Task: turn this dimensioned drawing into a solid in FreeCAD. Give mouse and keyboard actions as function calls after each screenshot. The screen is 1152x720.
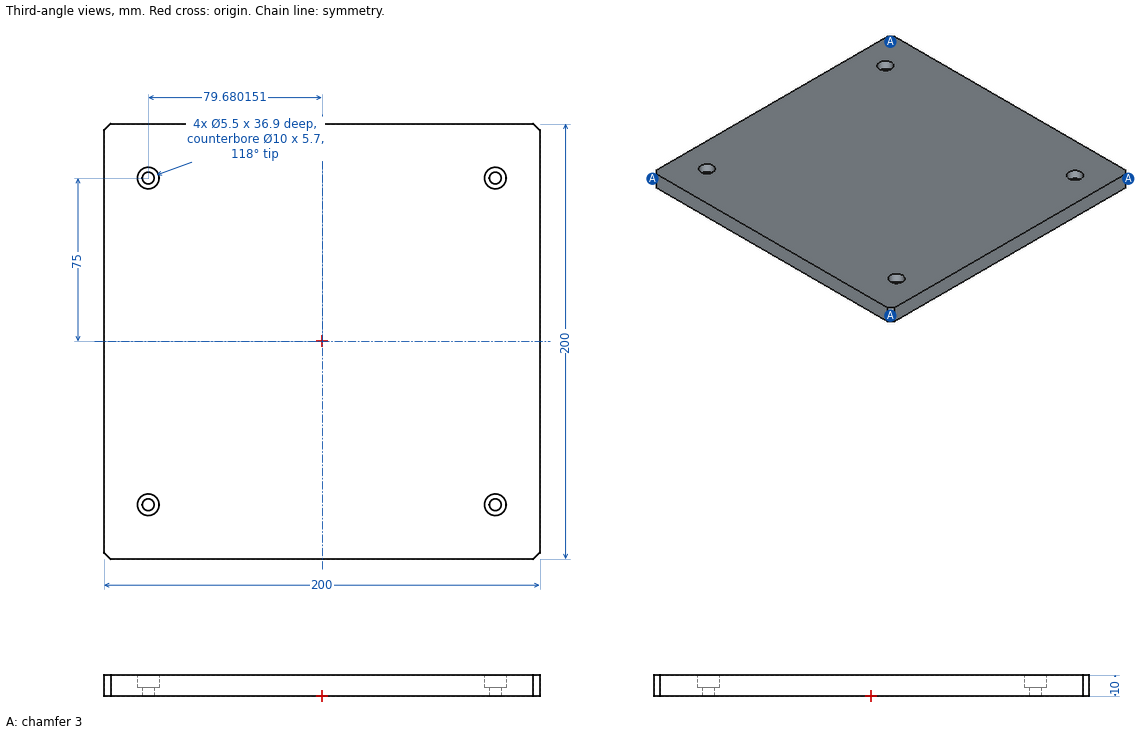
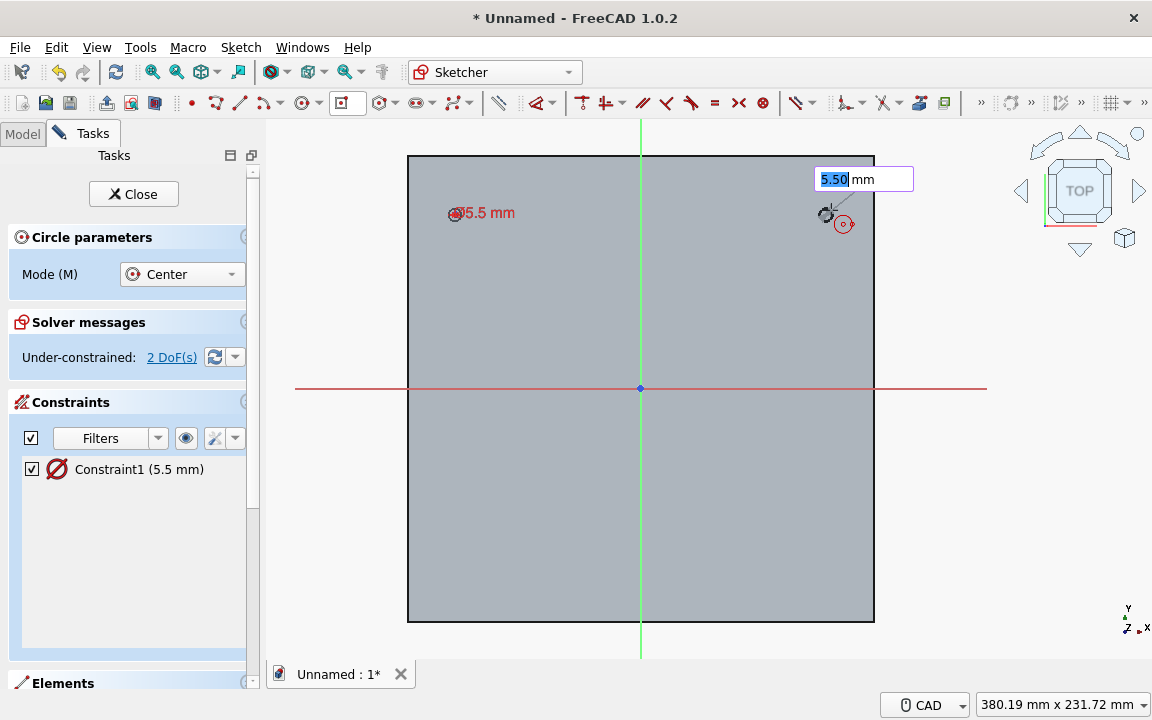
text(5.5)
key(Return)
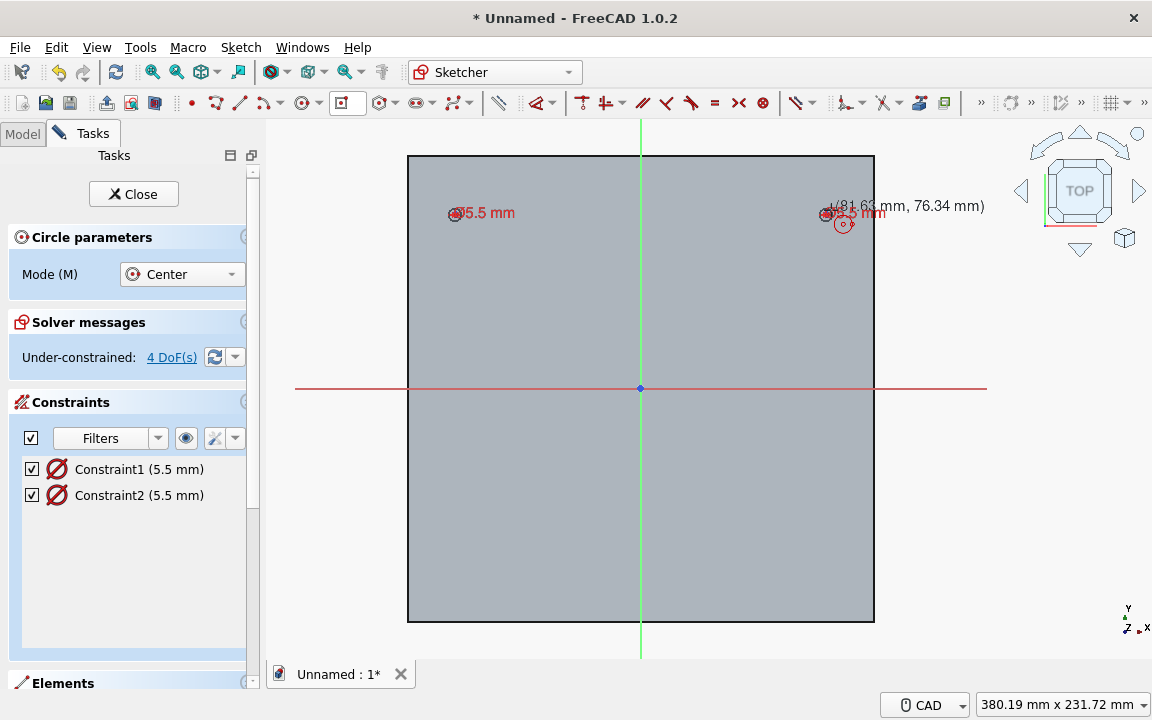
scroll(826, 564, up, 7)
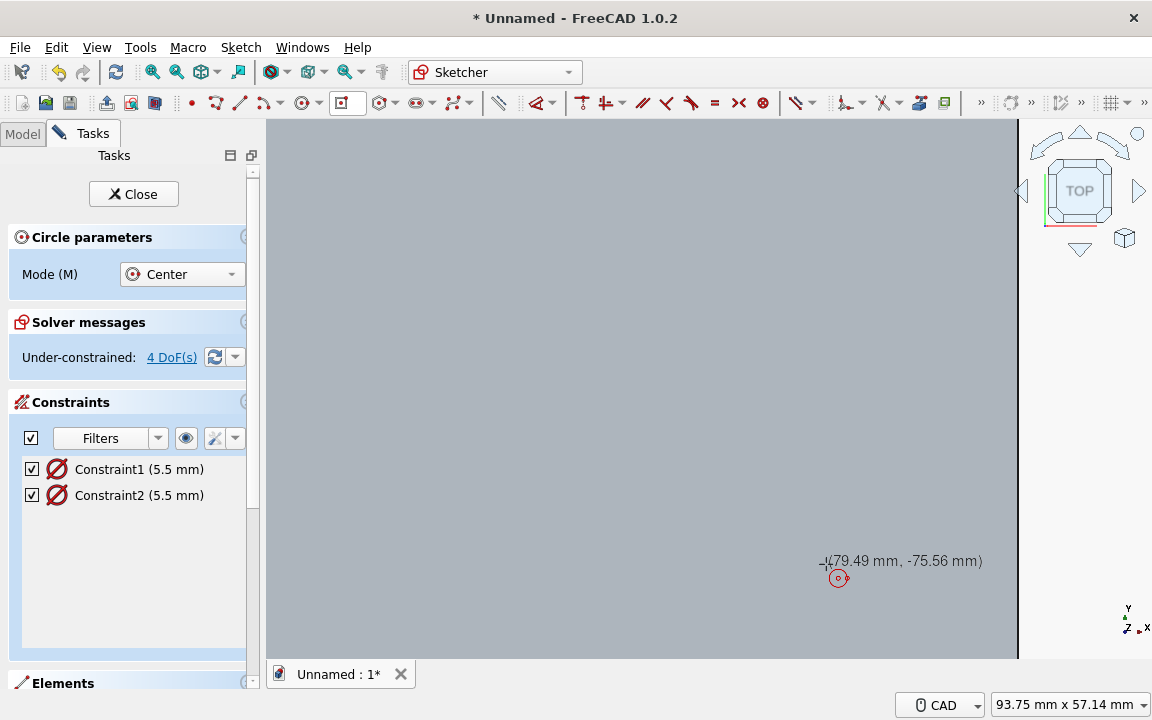
scroll(826, 565, down, 7)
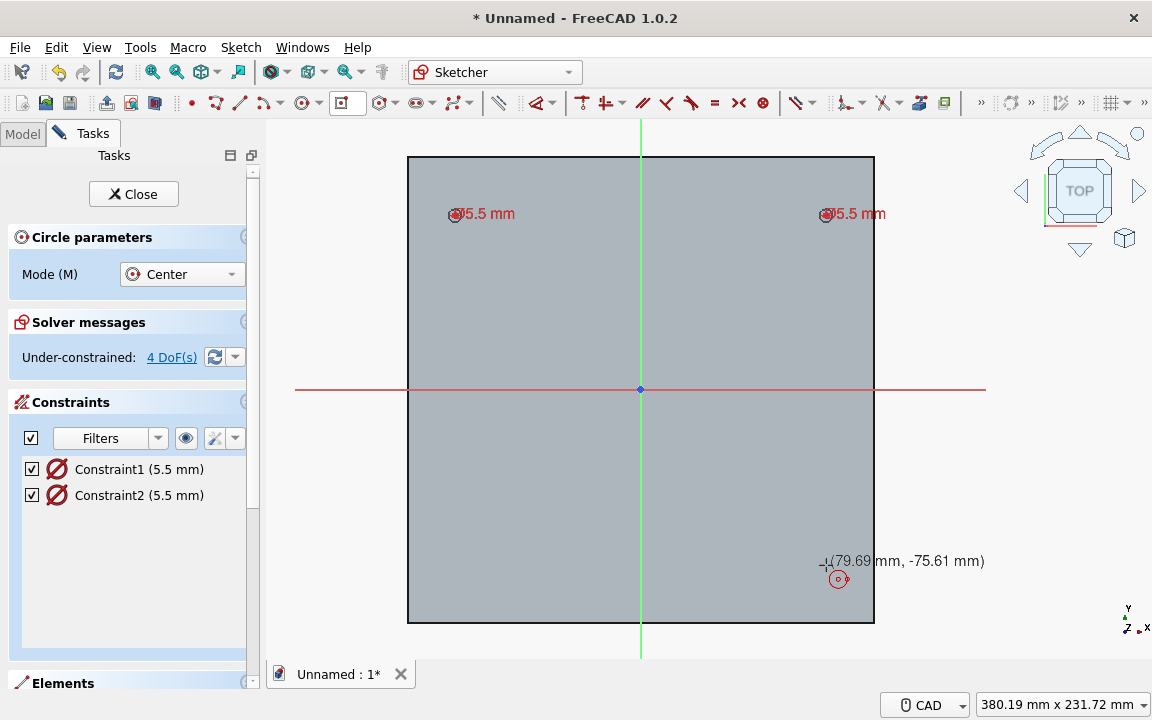
click(826, 564)
move(831, 560)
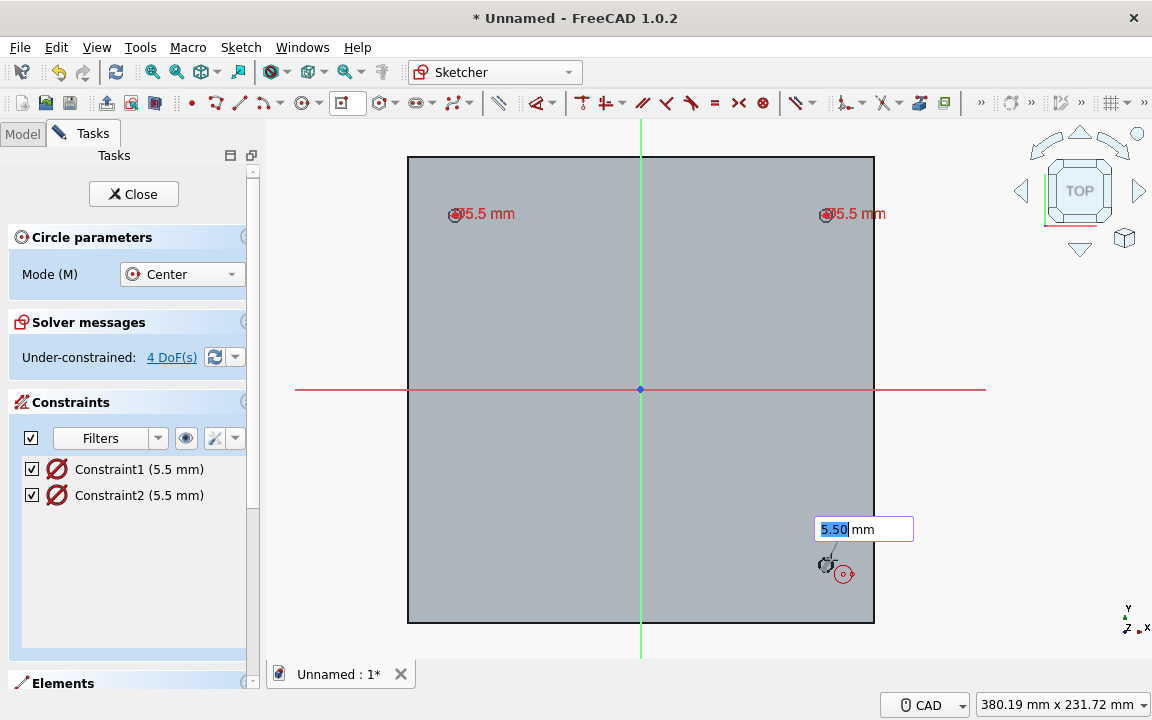
text(5.5)
key(Return)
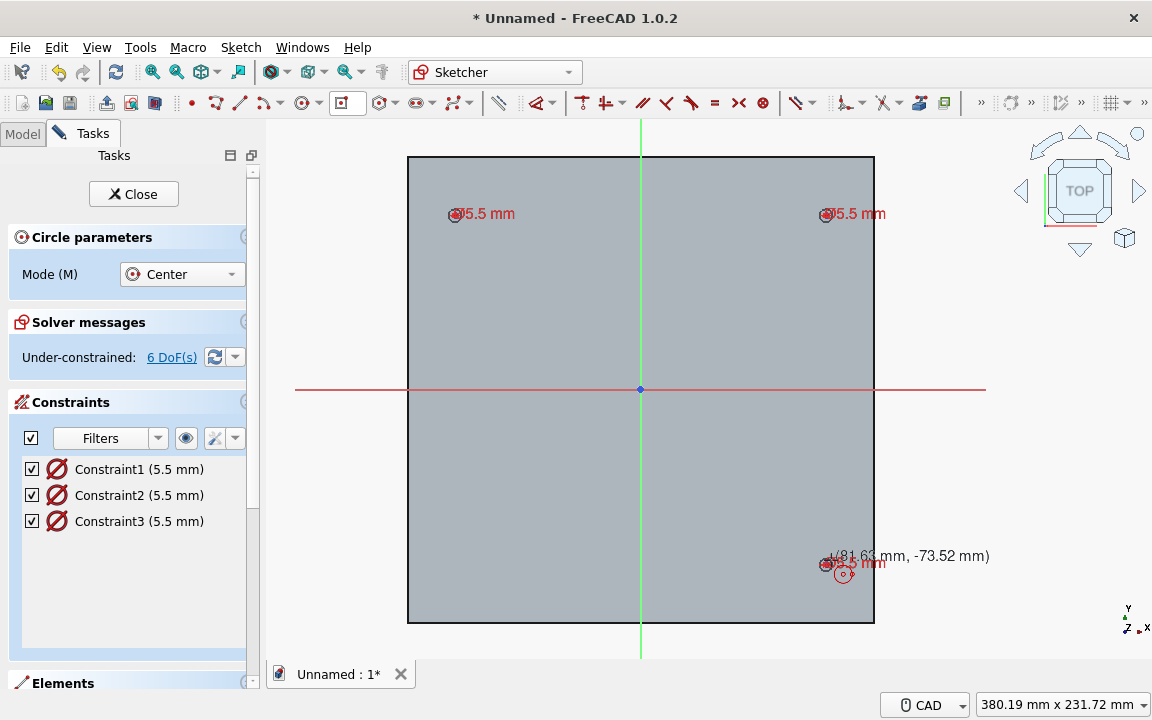
scroll(455, 564, up, 7)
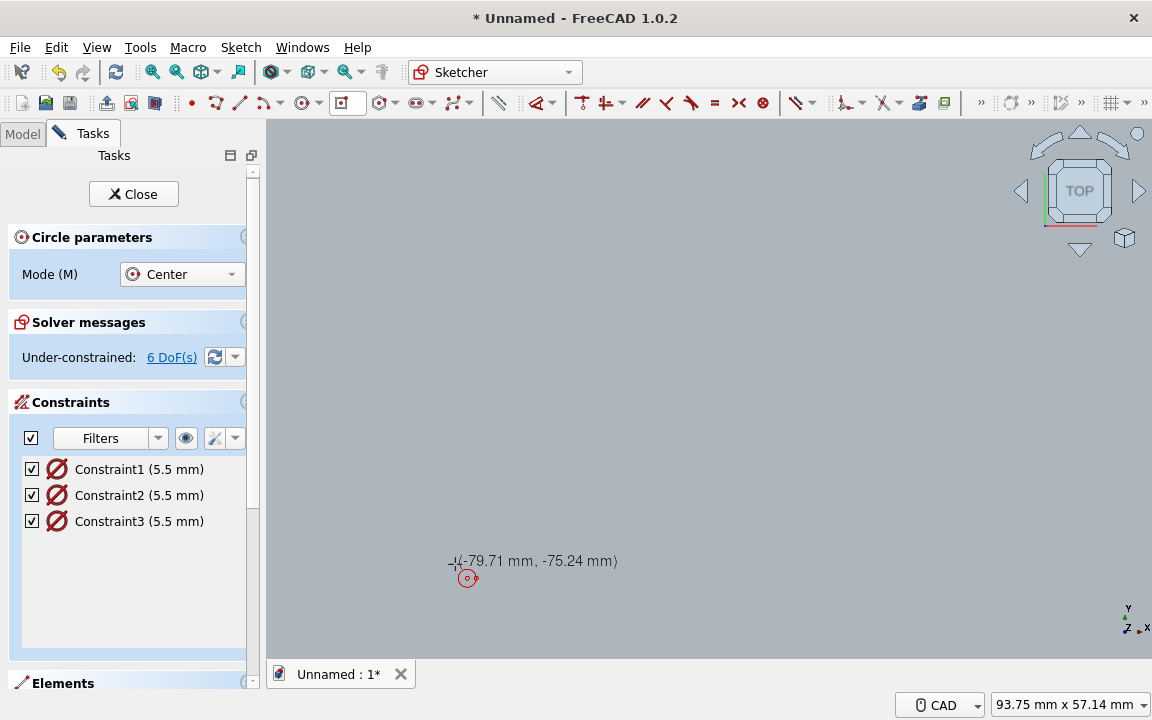
scroll(455, 564, down, 7)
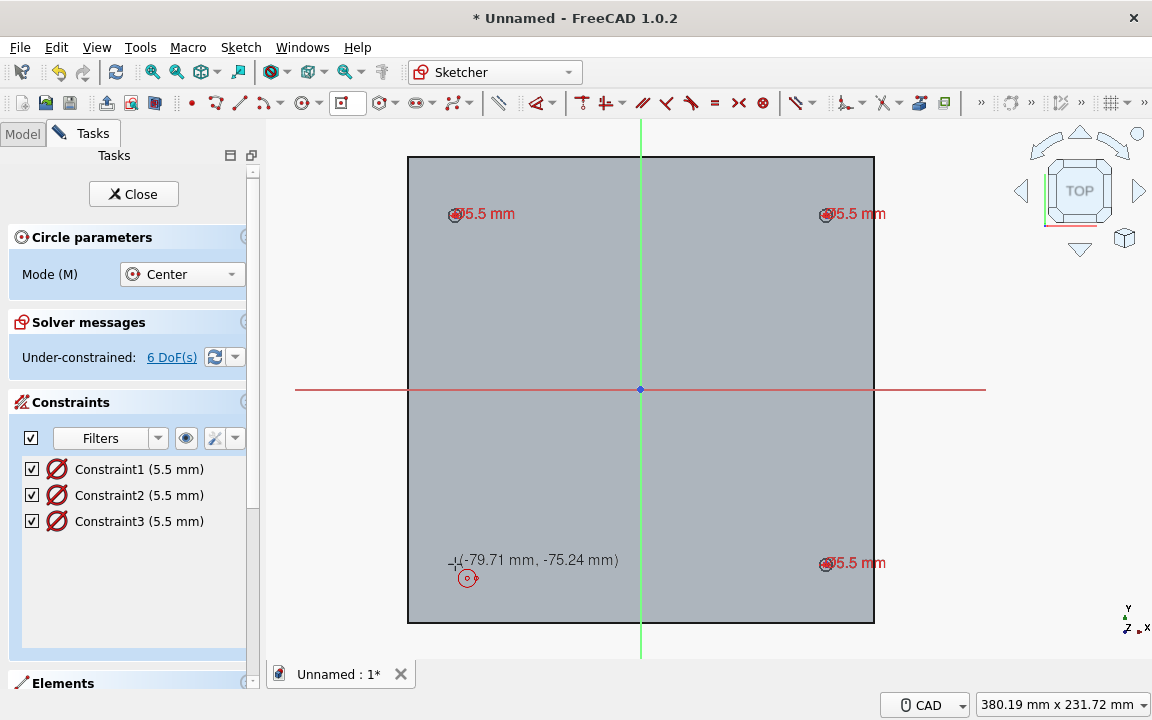
click(455, 564)
move(460, 560)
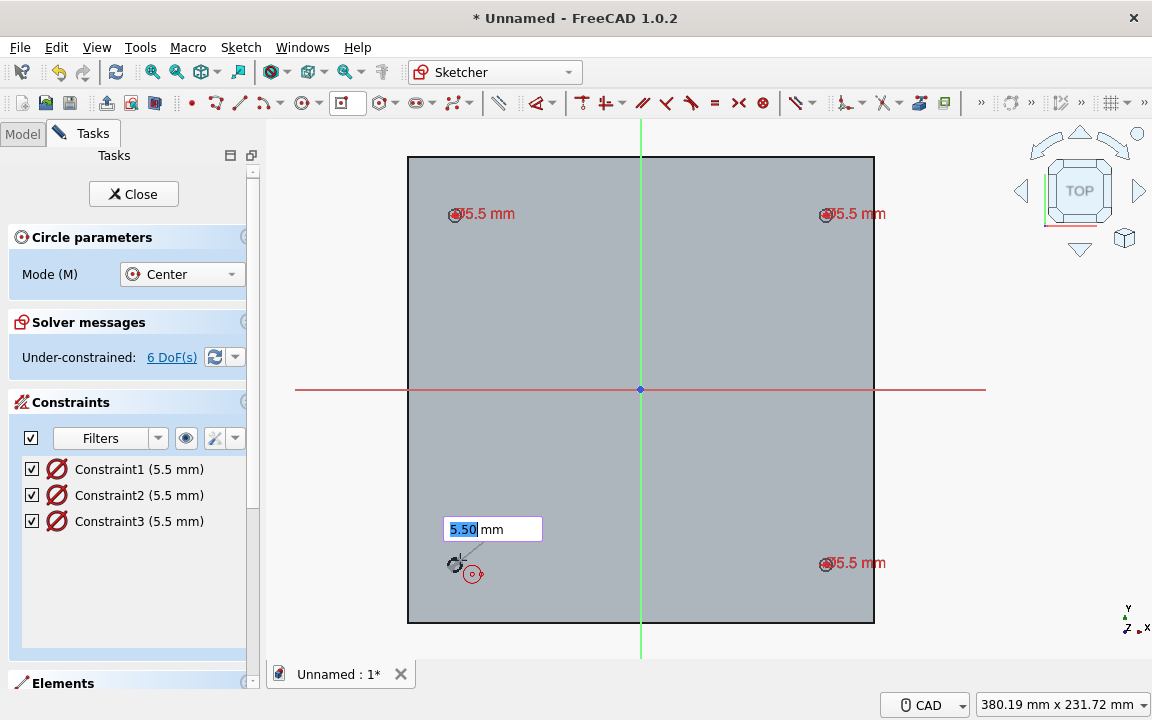
text(5.5)
key(Return)
key(Escape)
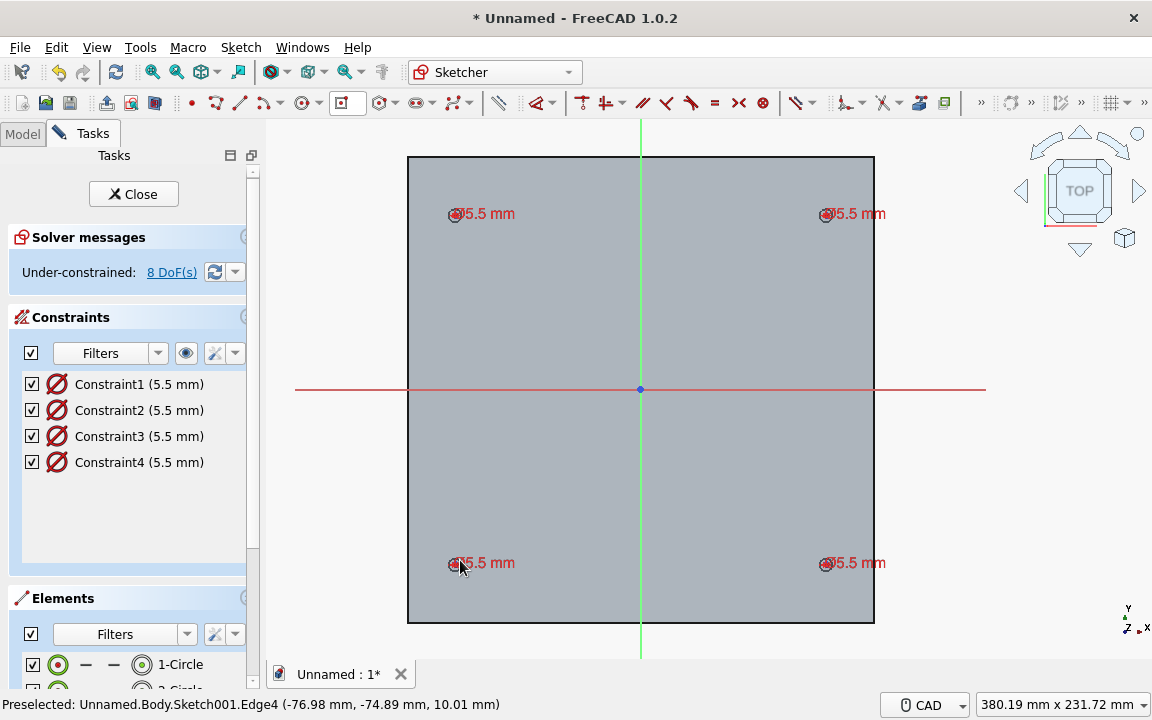
click(455, 216)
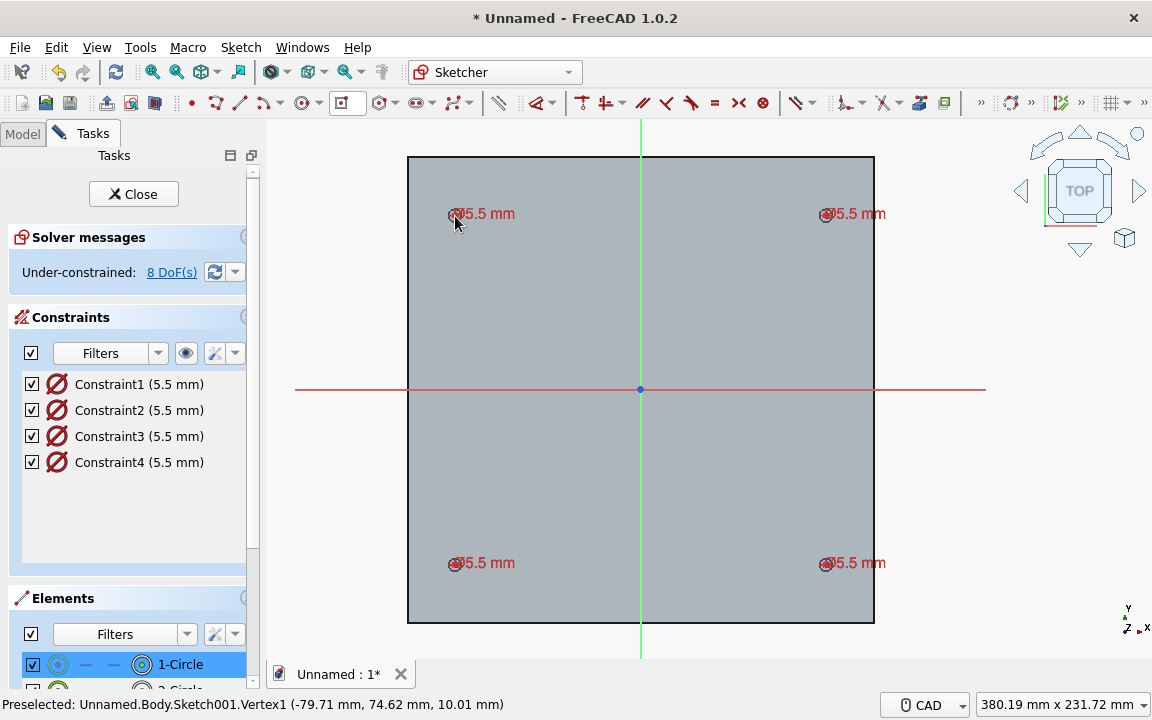
click(826, 216)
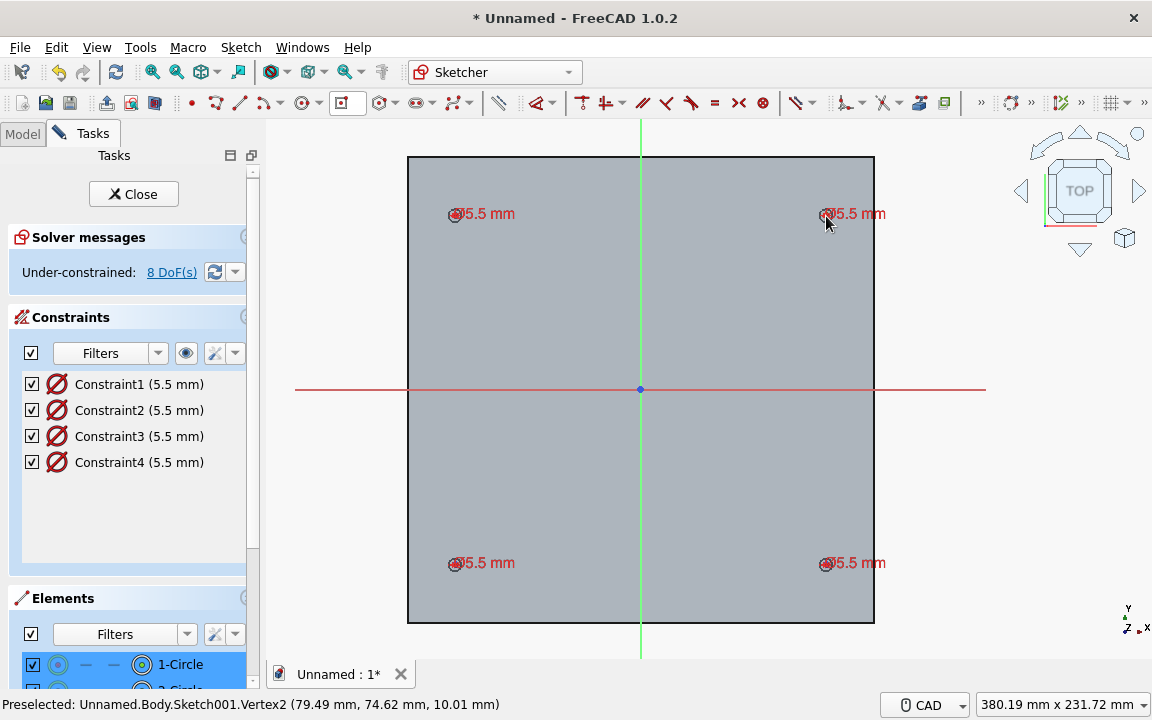
click(641, 596)